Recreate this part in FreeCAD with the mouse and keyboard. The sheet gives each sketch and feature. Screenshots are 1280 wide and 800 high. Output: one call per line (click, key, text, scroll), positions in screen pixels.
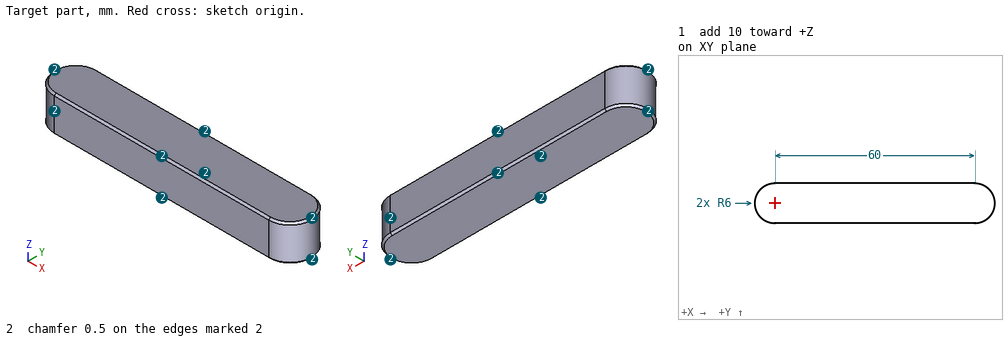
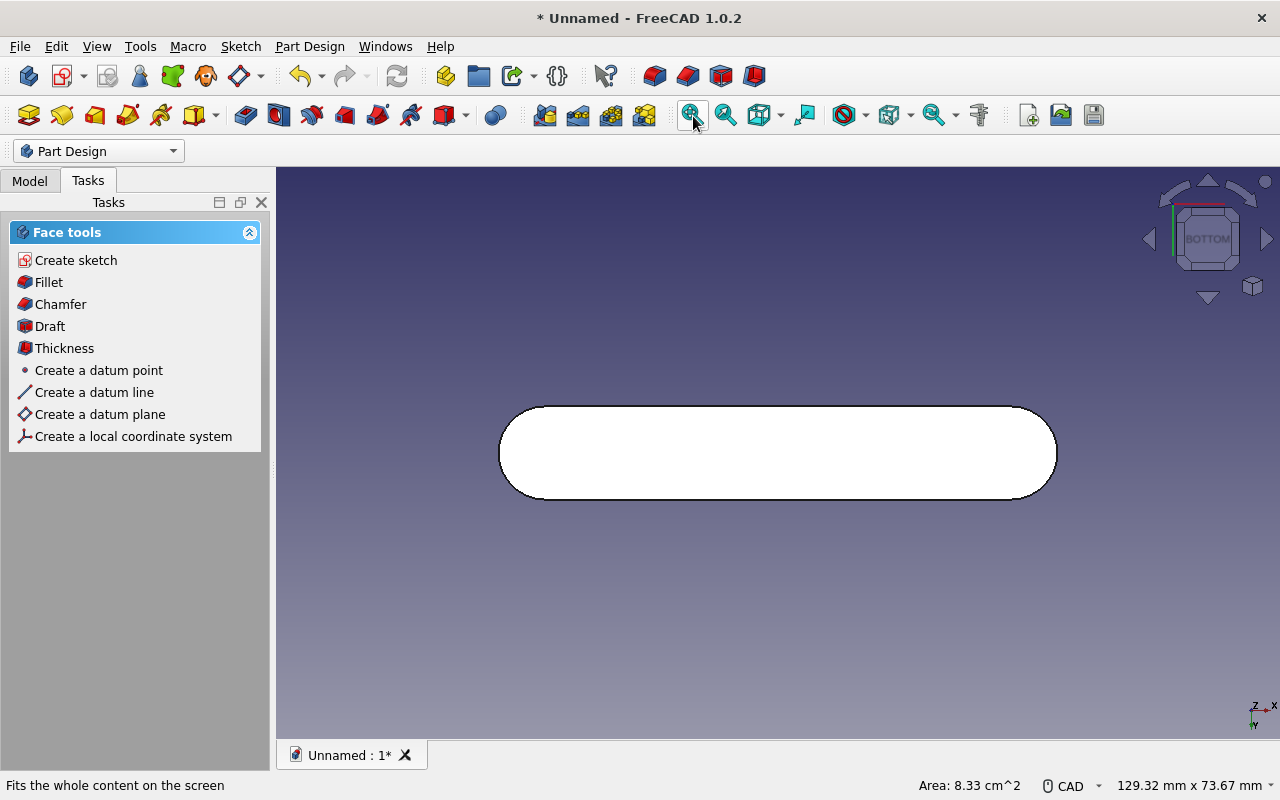
click(938, 452, ctrl)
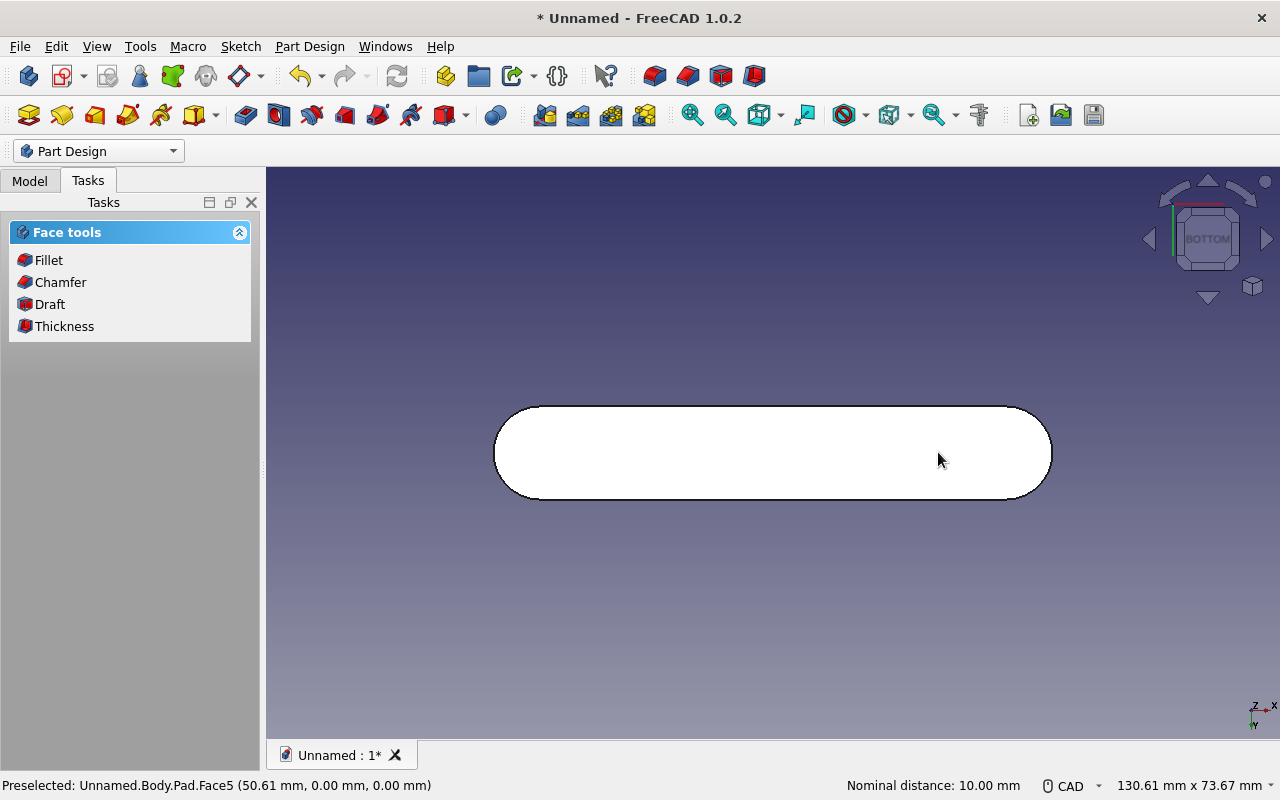
click(688, 76)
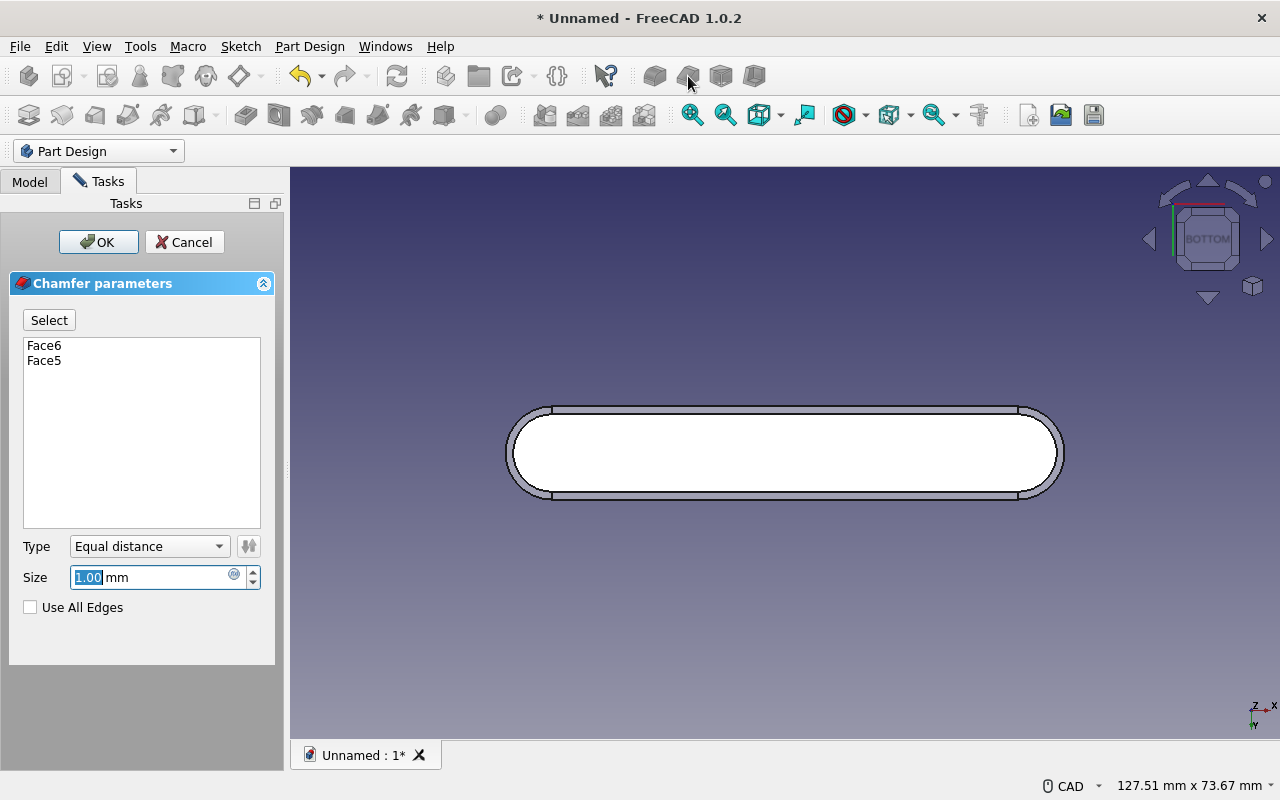
text(0.5)
key(Tab)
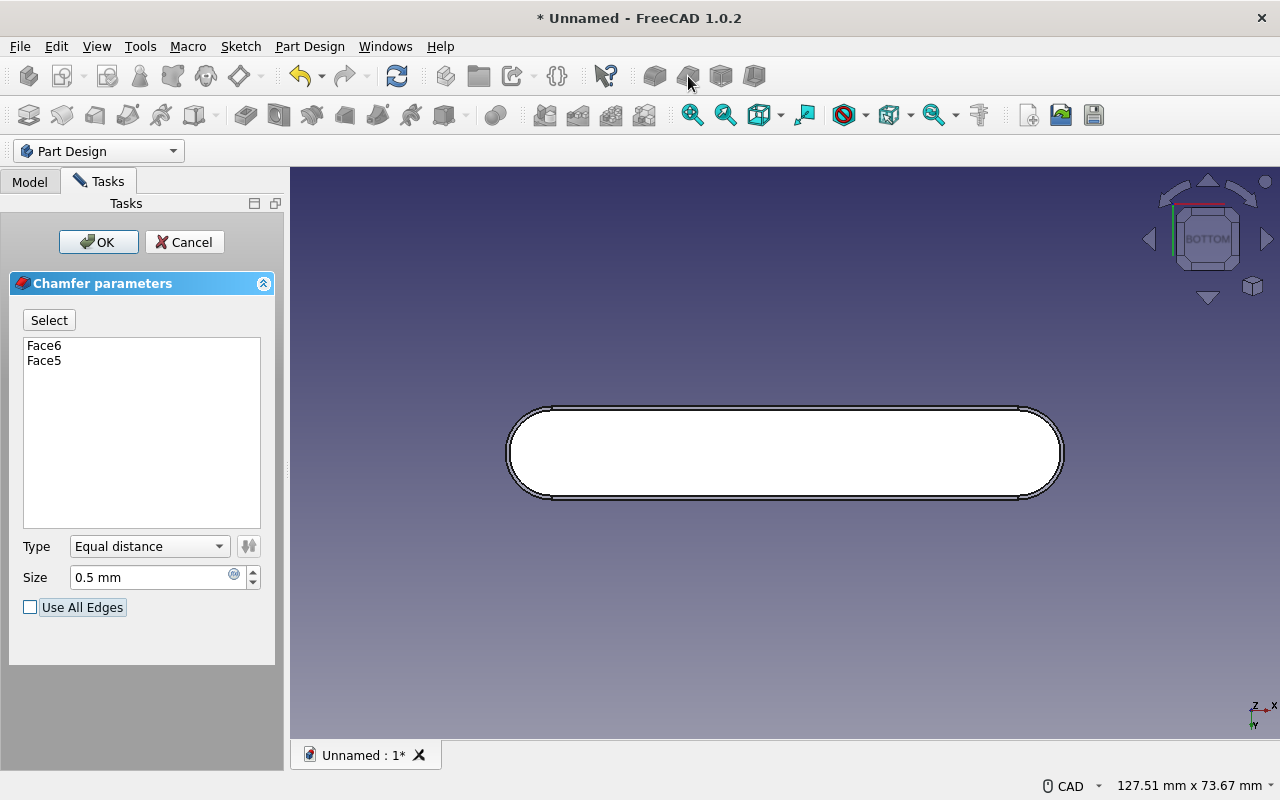
click(99, 242)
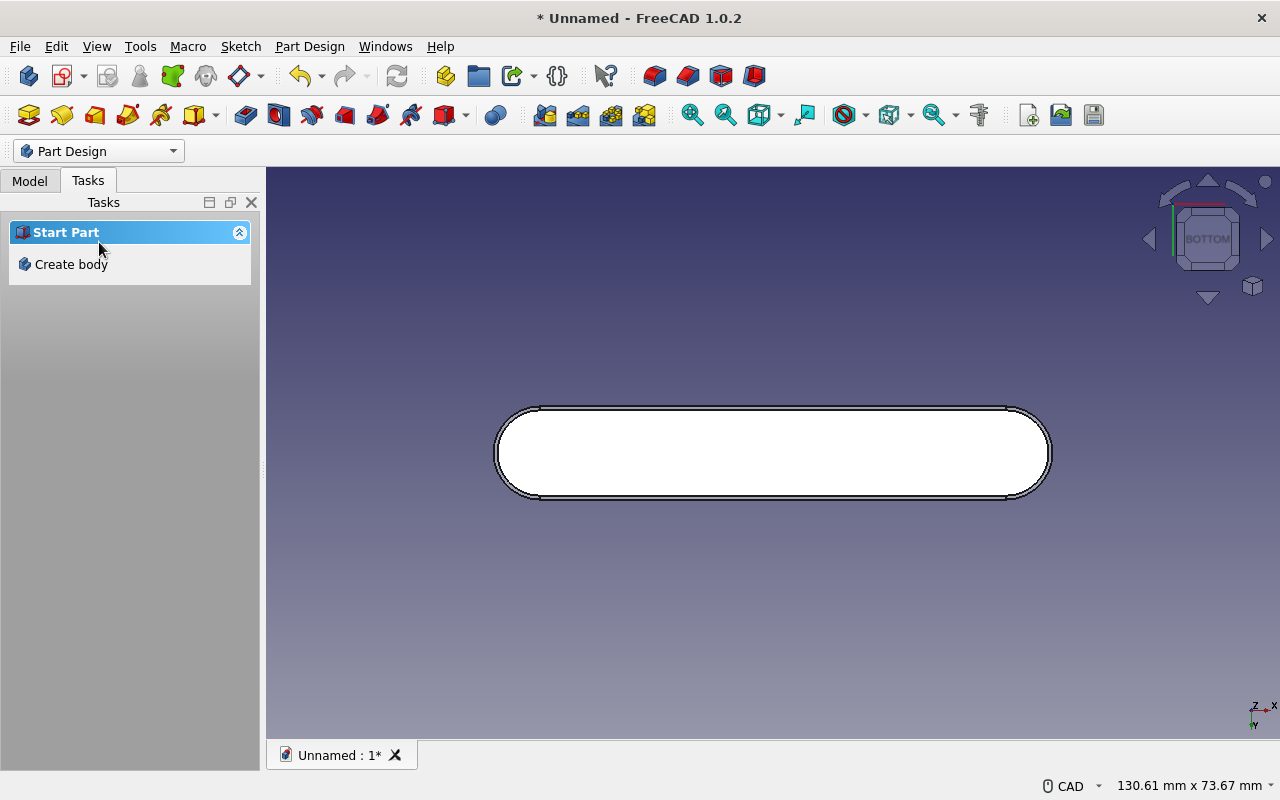
key(0)